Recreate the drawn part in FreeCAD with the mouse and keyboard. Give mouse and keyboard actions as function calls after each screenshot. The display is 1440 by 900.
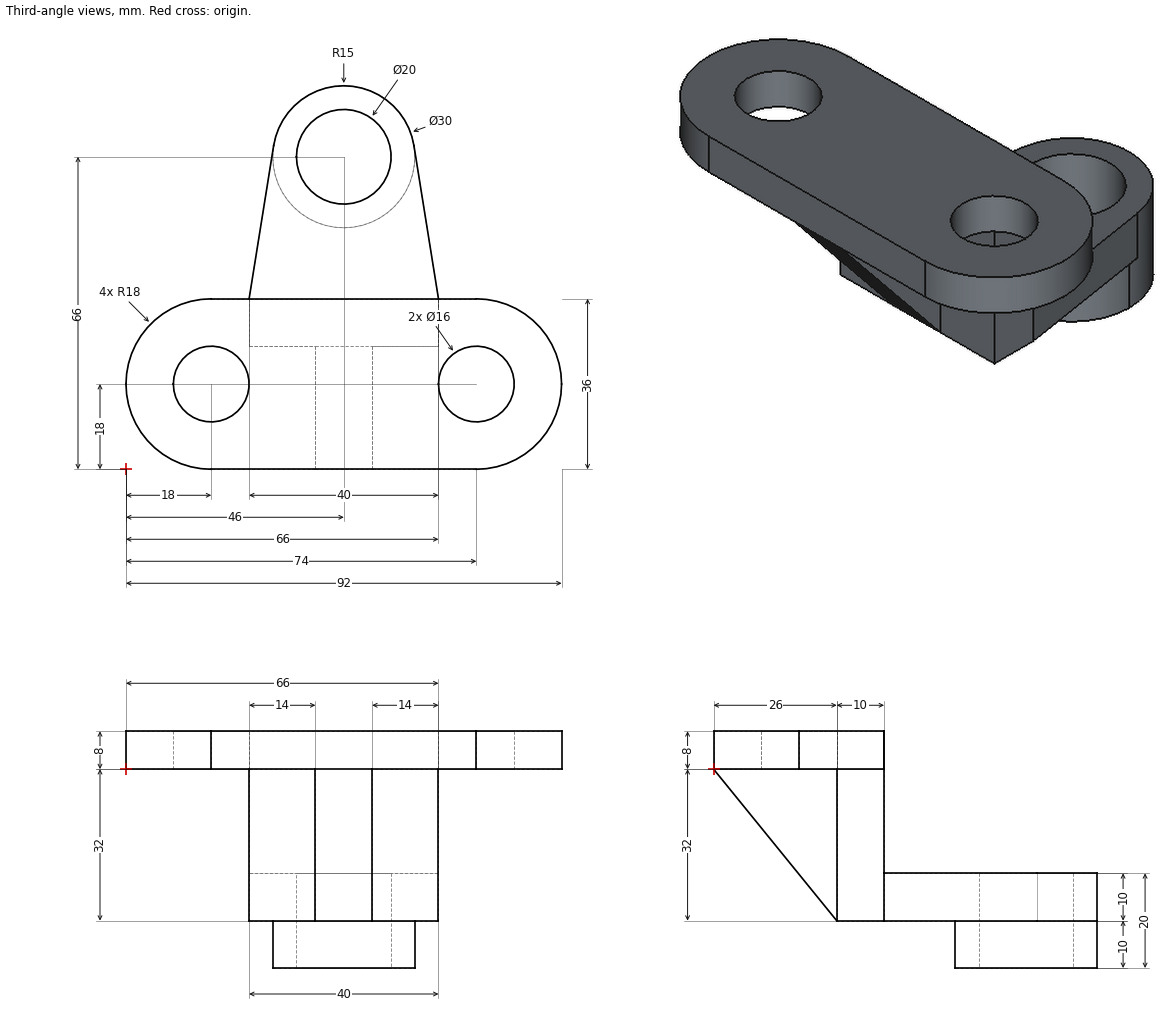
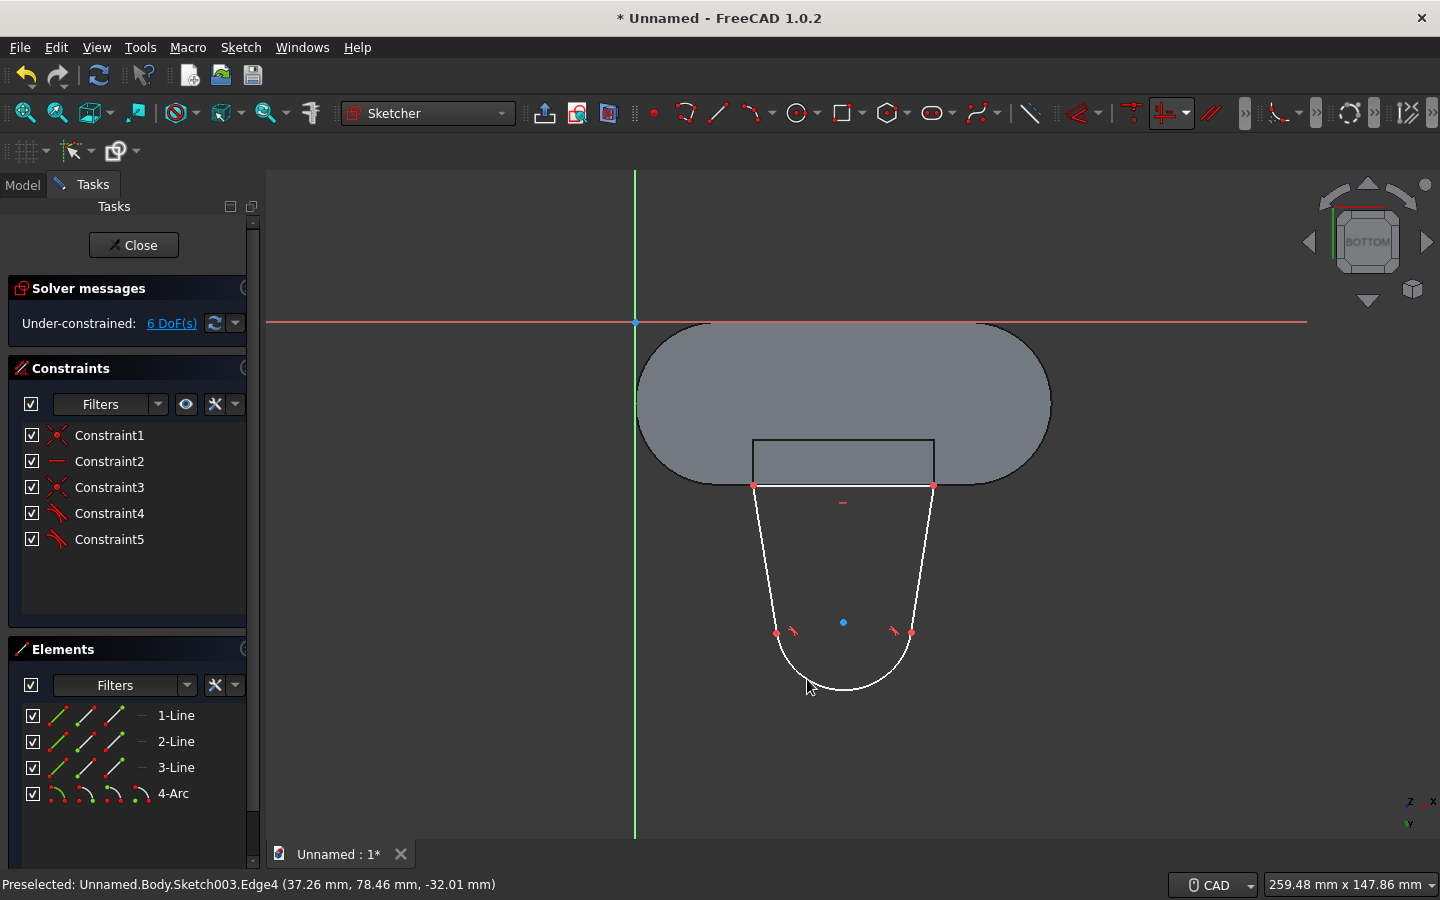
click(1078, 114)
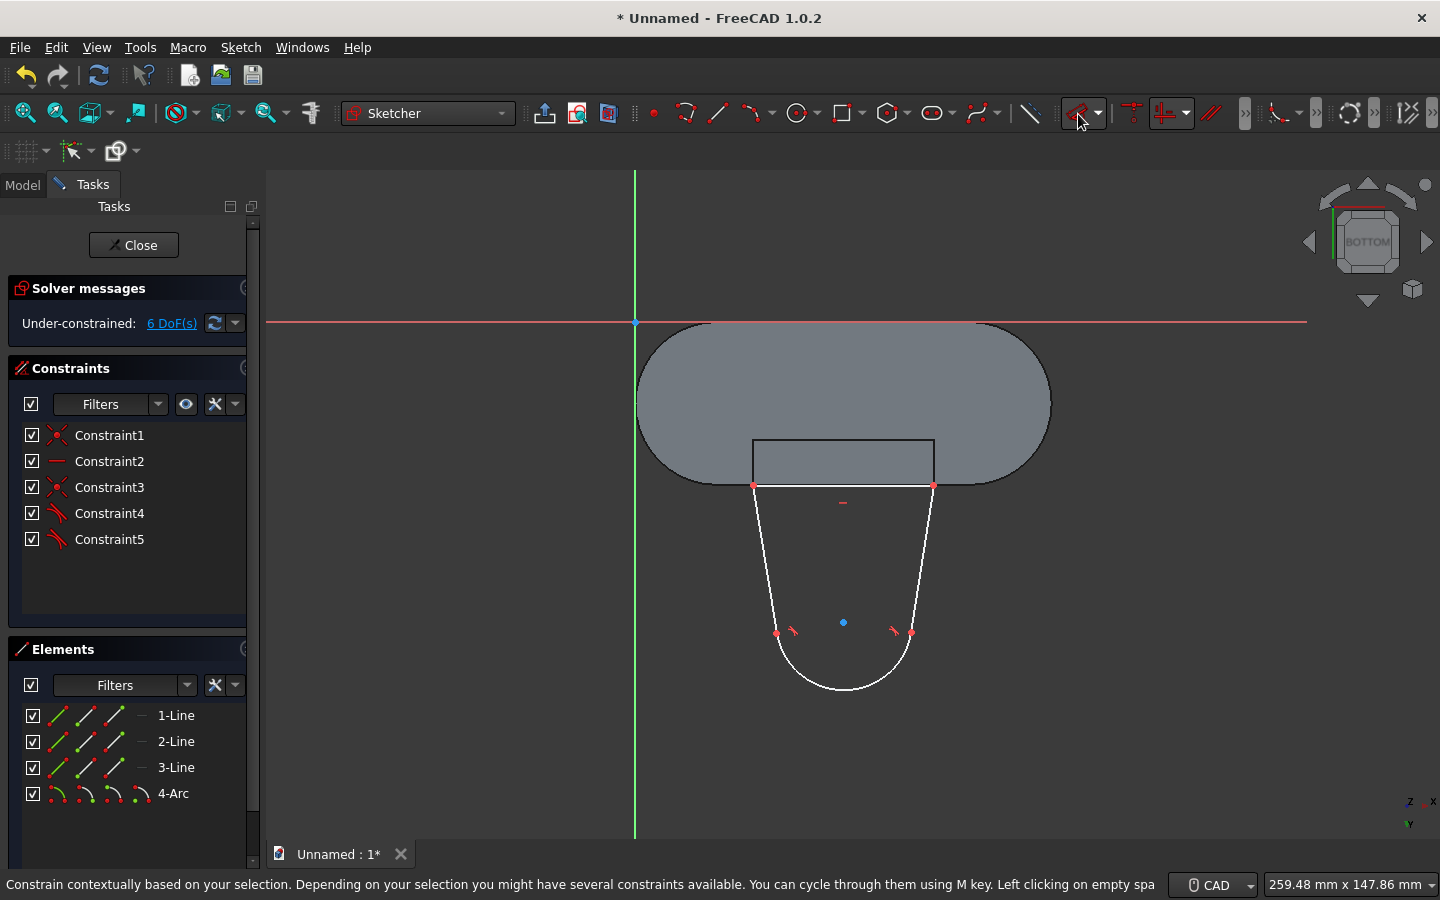
click(808, 680)
click(791, 707)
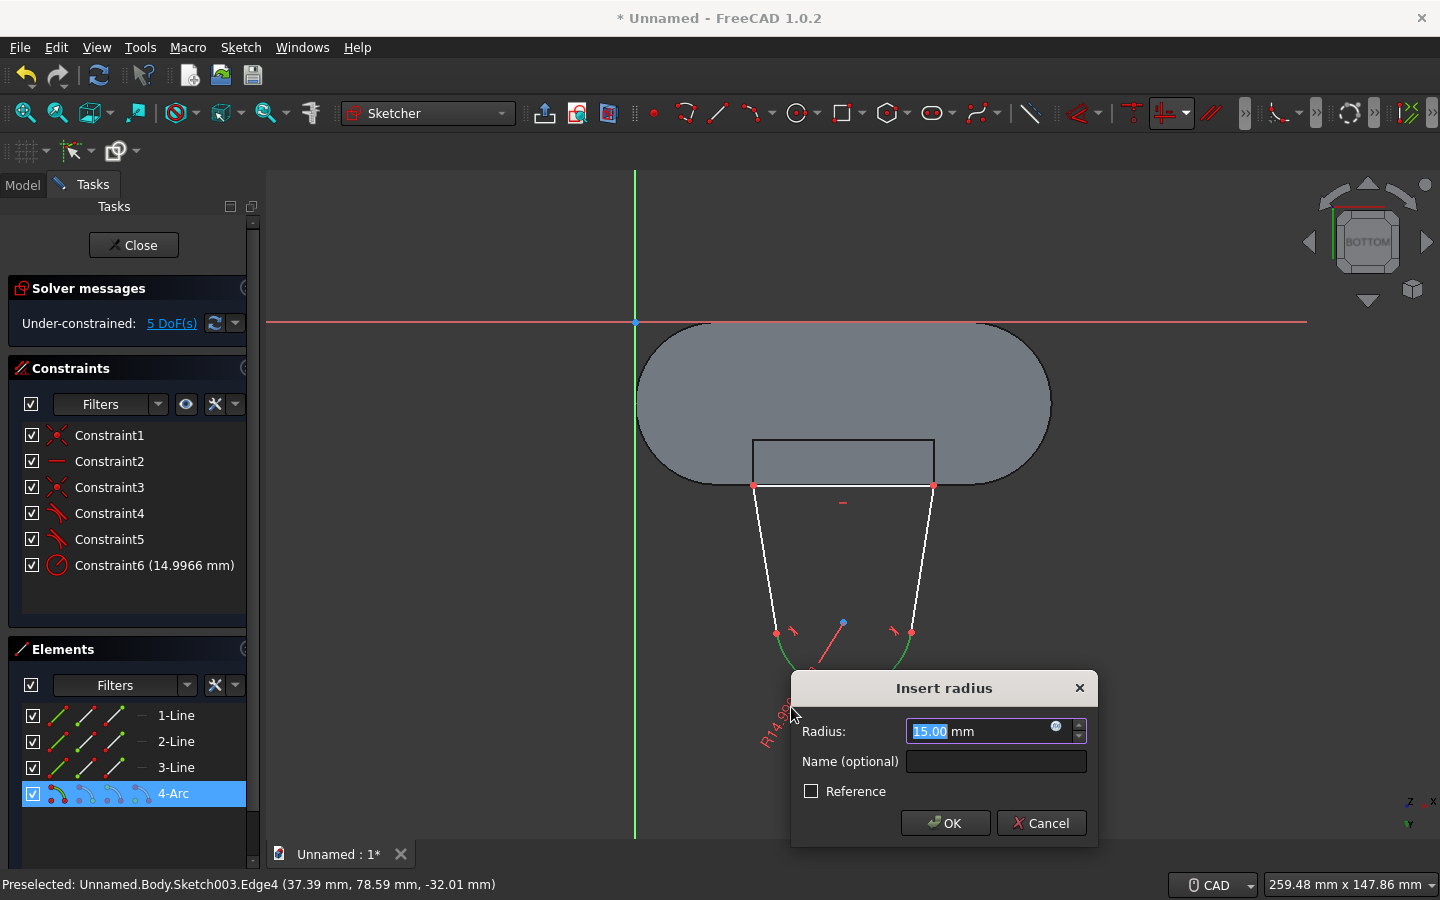
text(15)
key(Return)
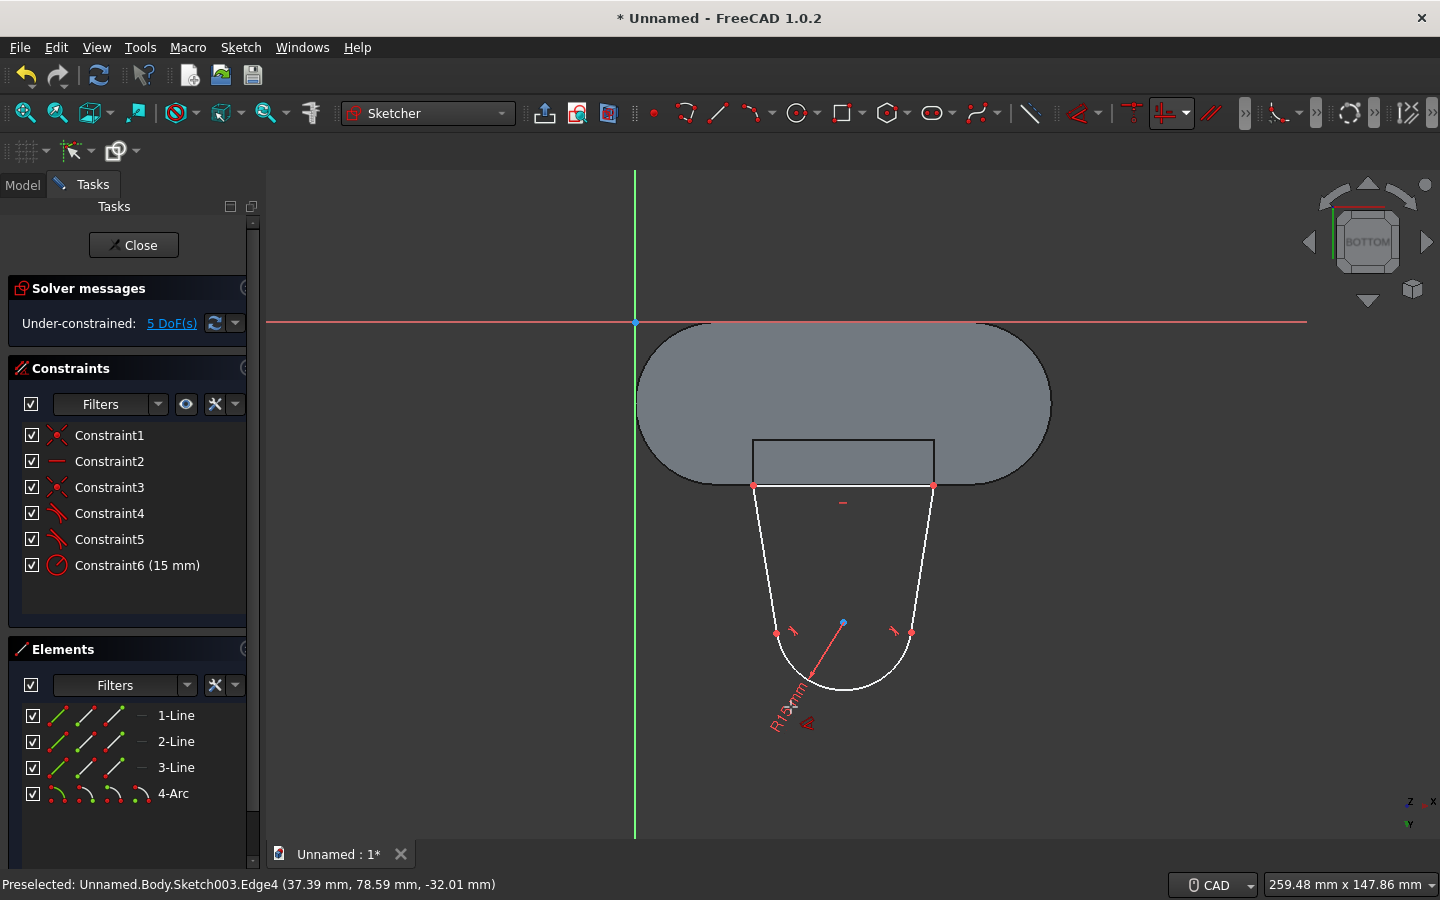
click(880, 486)
click(844, 452)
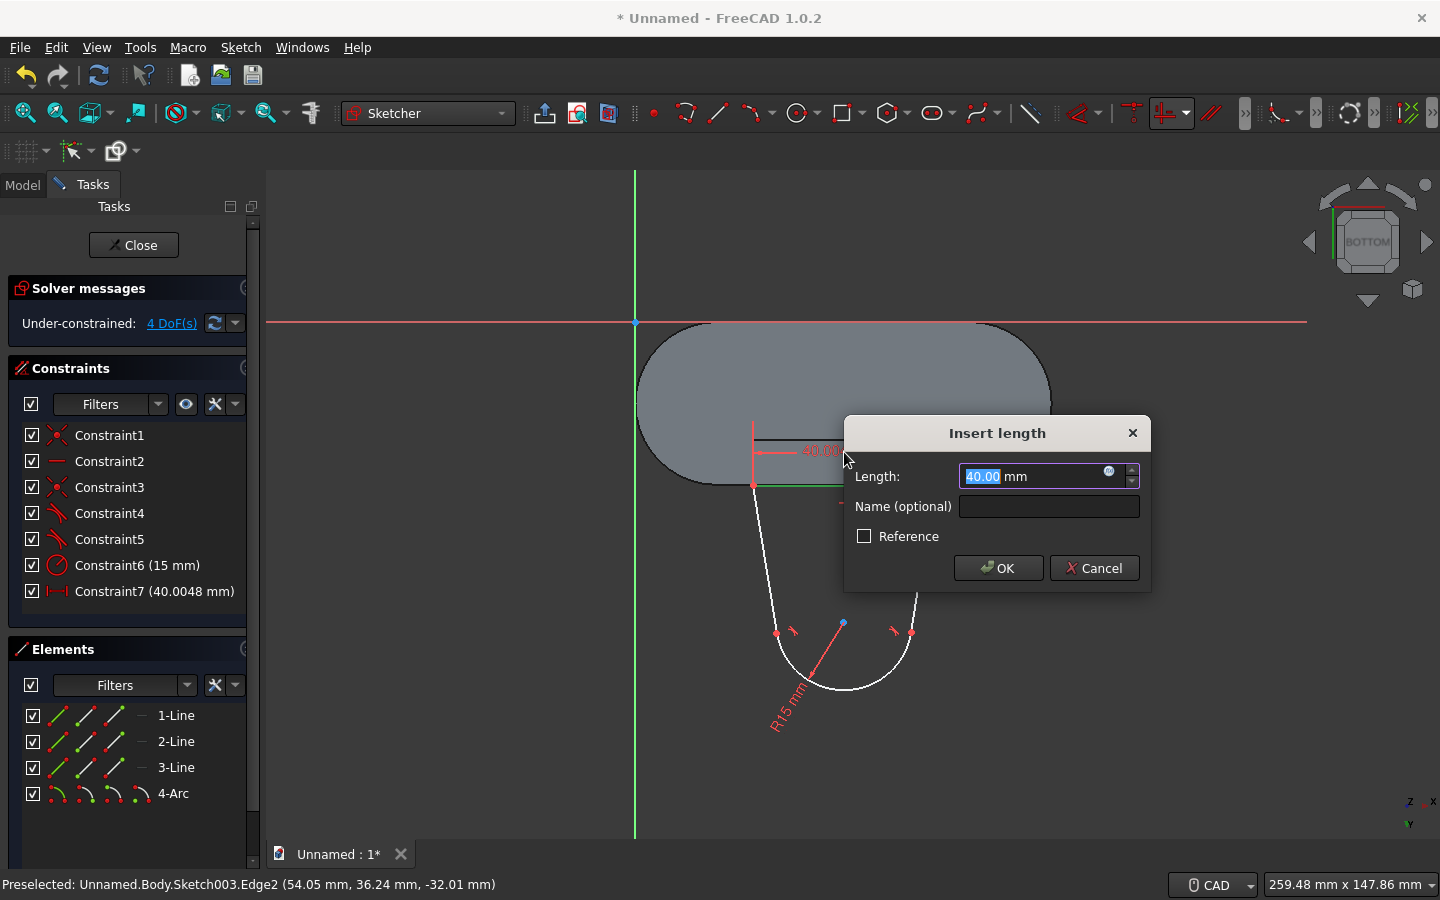
text(40)
key(Return)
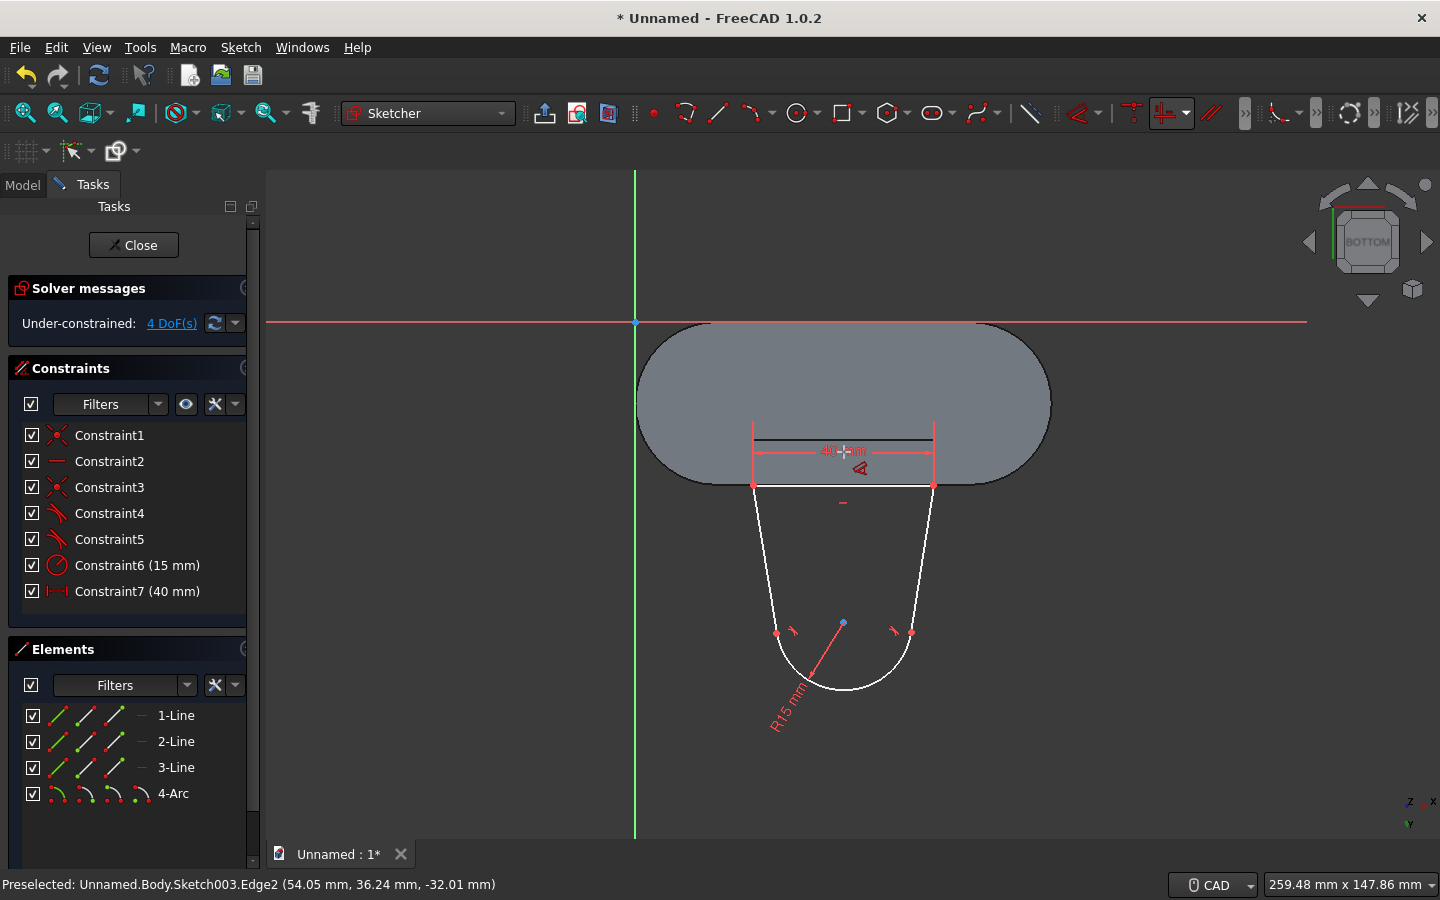
click(934, 486)
click(785, 288)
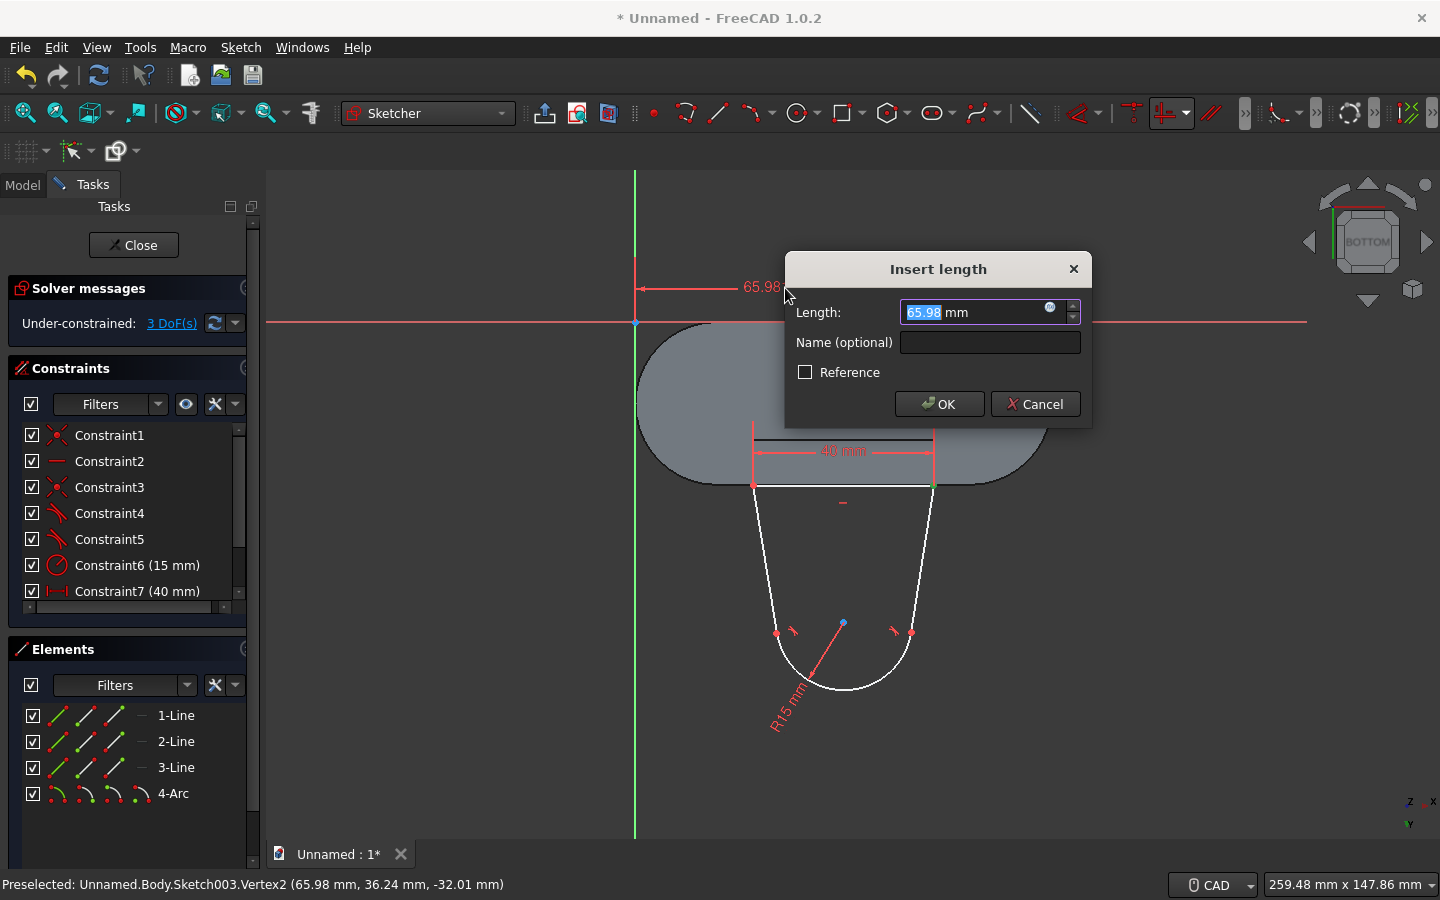
text(66)
key(Return)